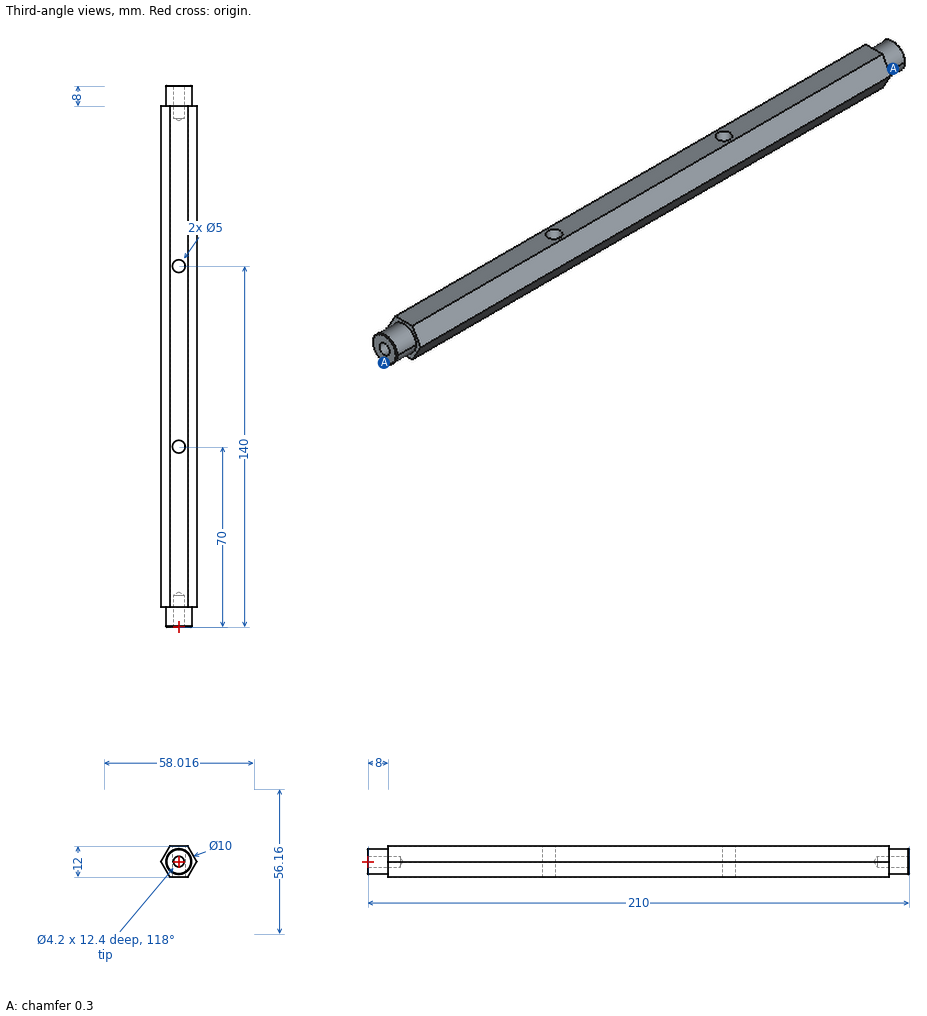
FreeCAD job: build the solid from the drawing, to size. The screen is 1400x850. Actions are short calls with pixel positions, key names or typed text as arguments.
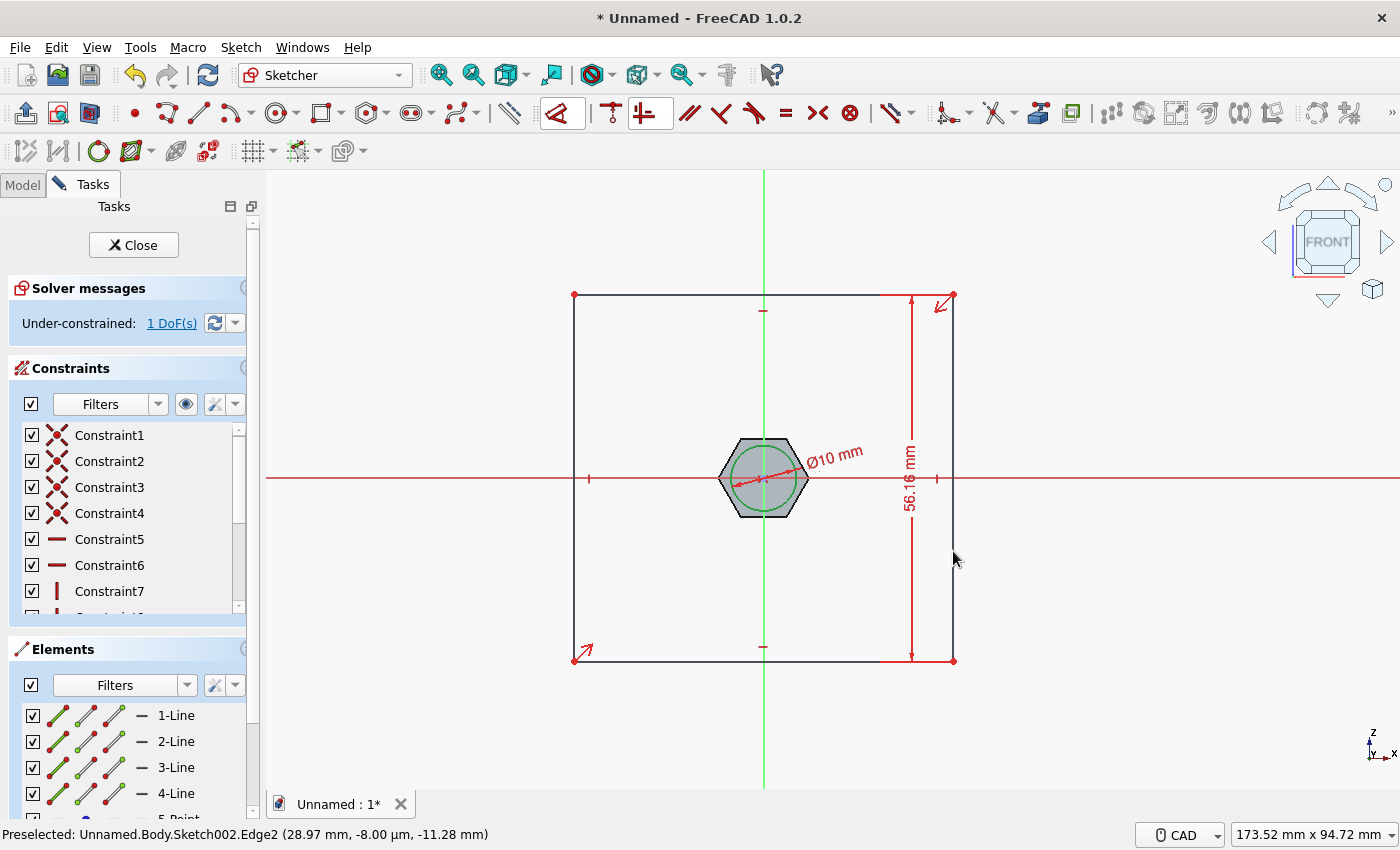
click(688, 662)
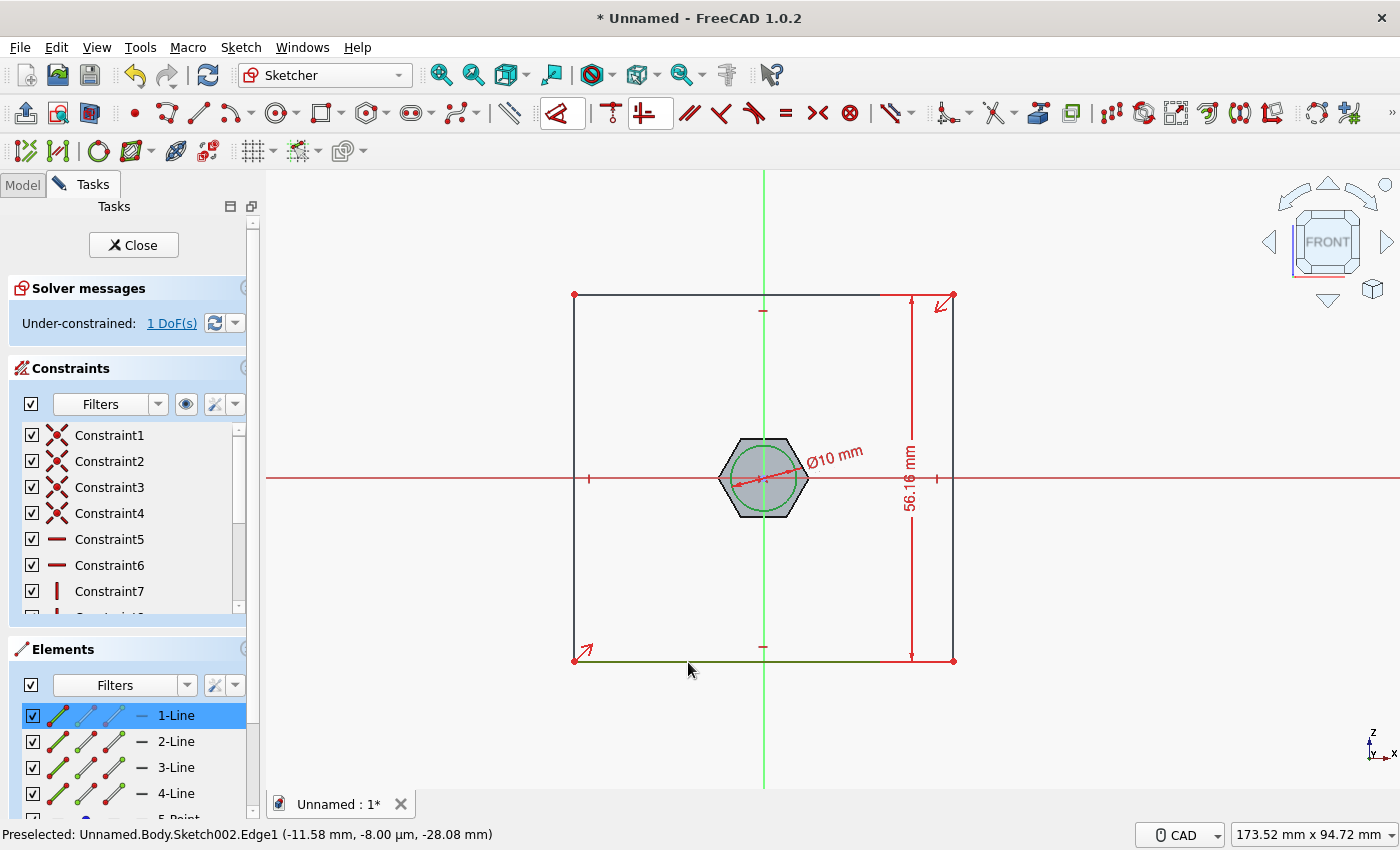
key(l)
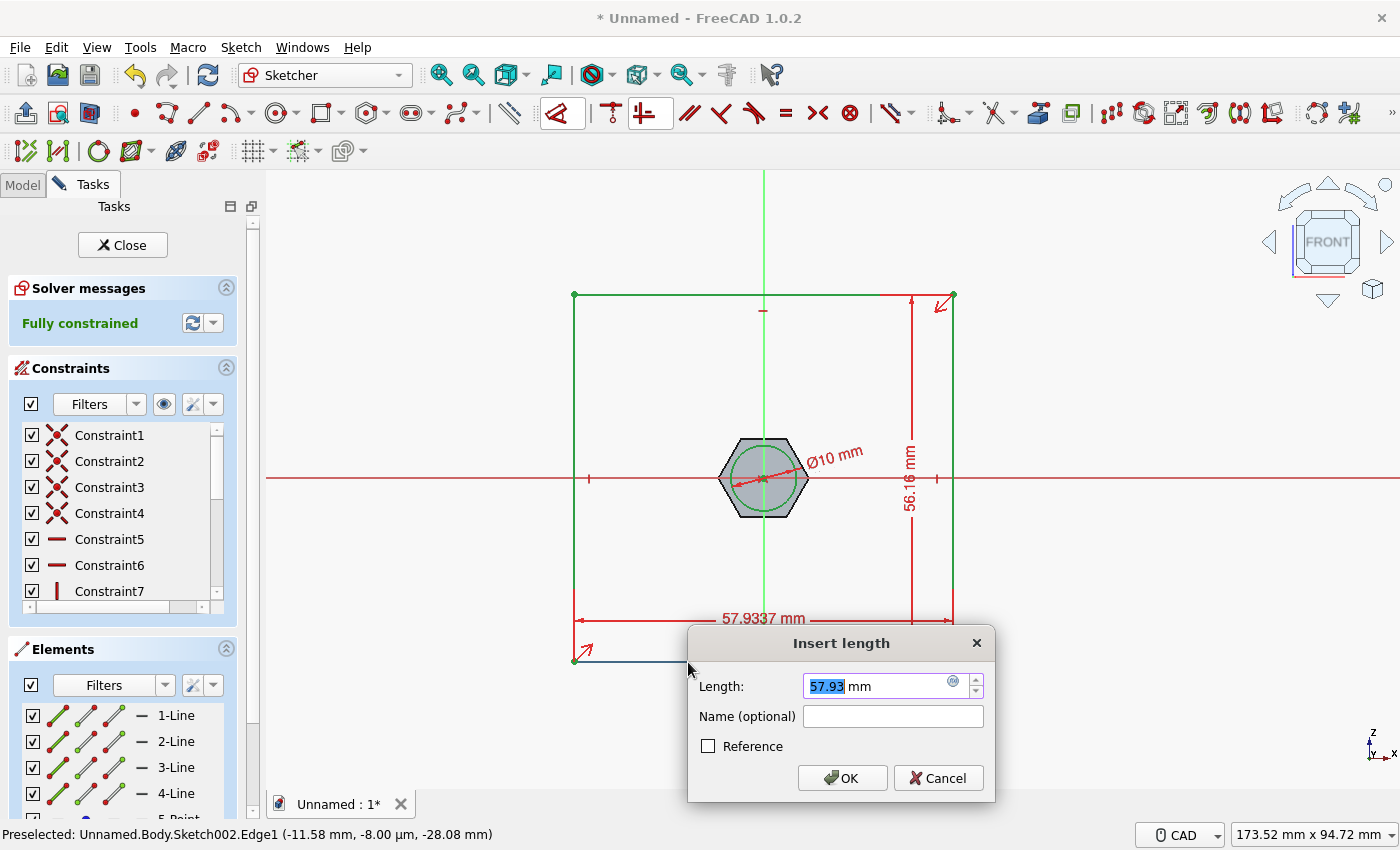
text(58.016)
key(Return)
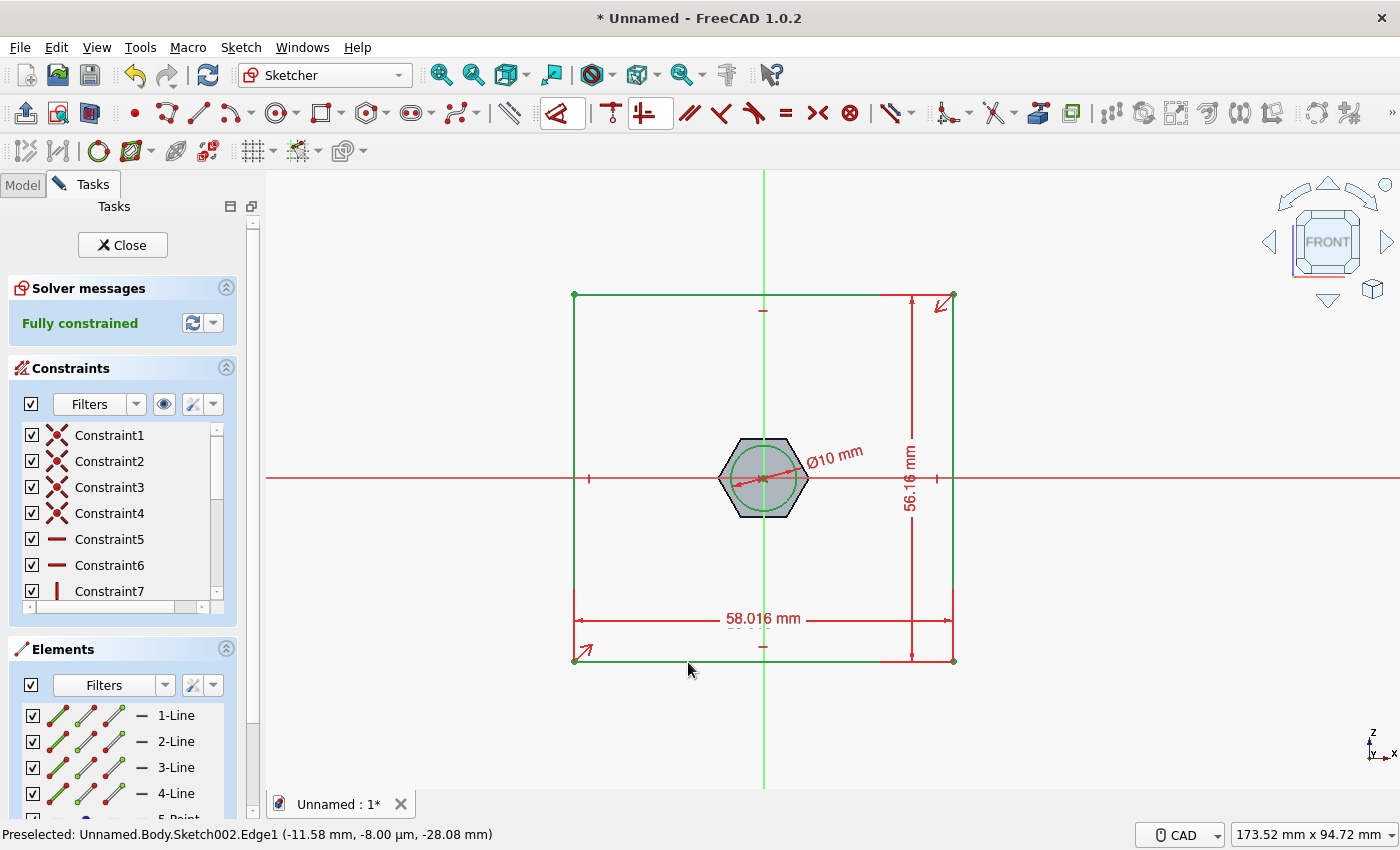
click(123, 245)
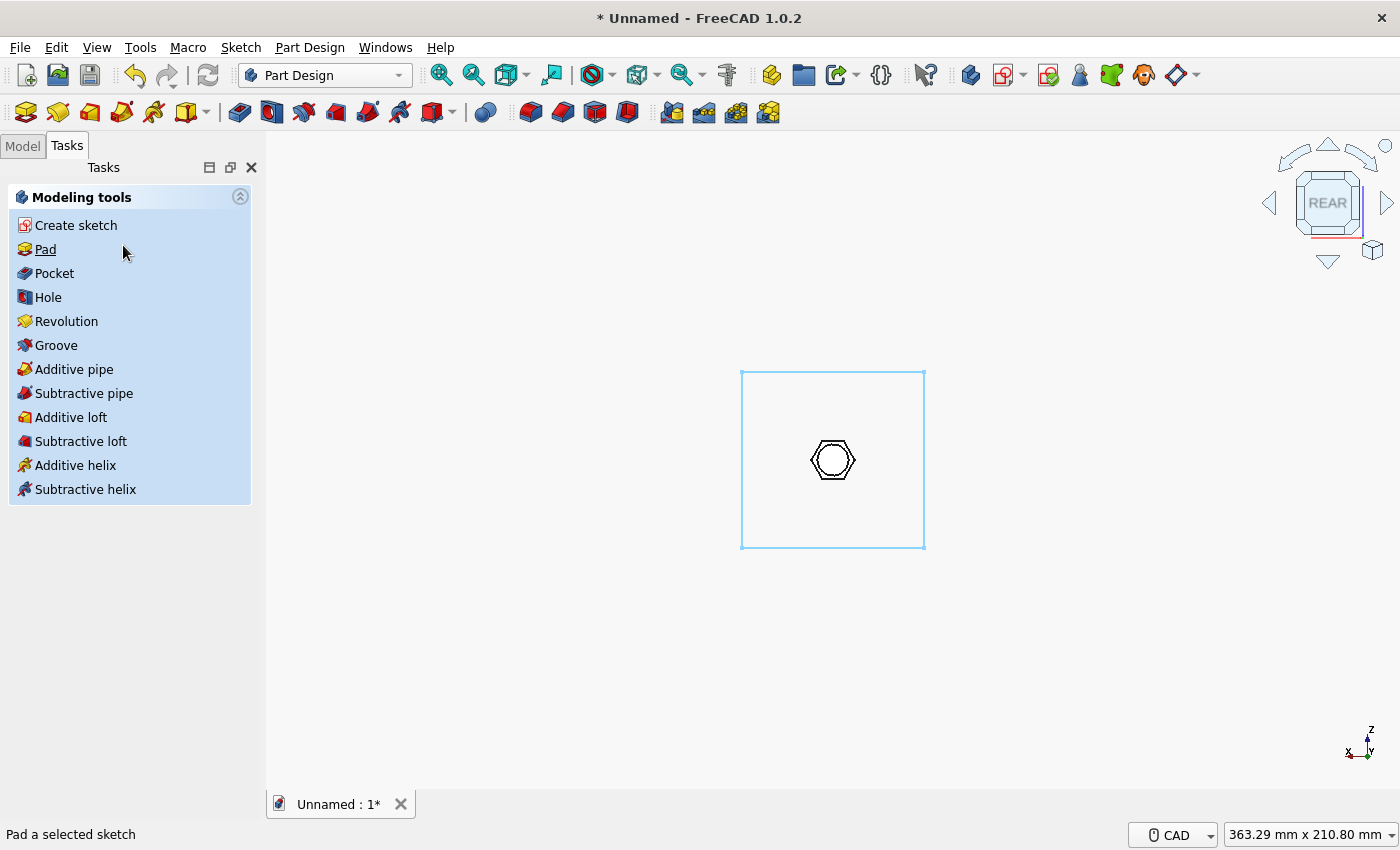
click(240, 112)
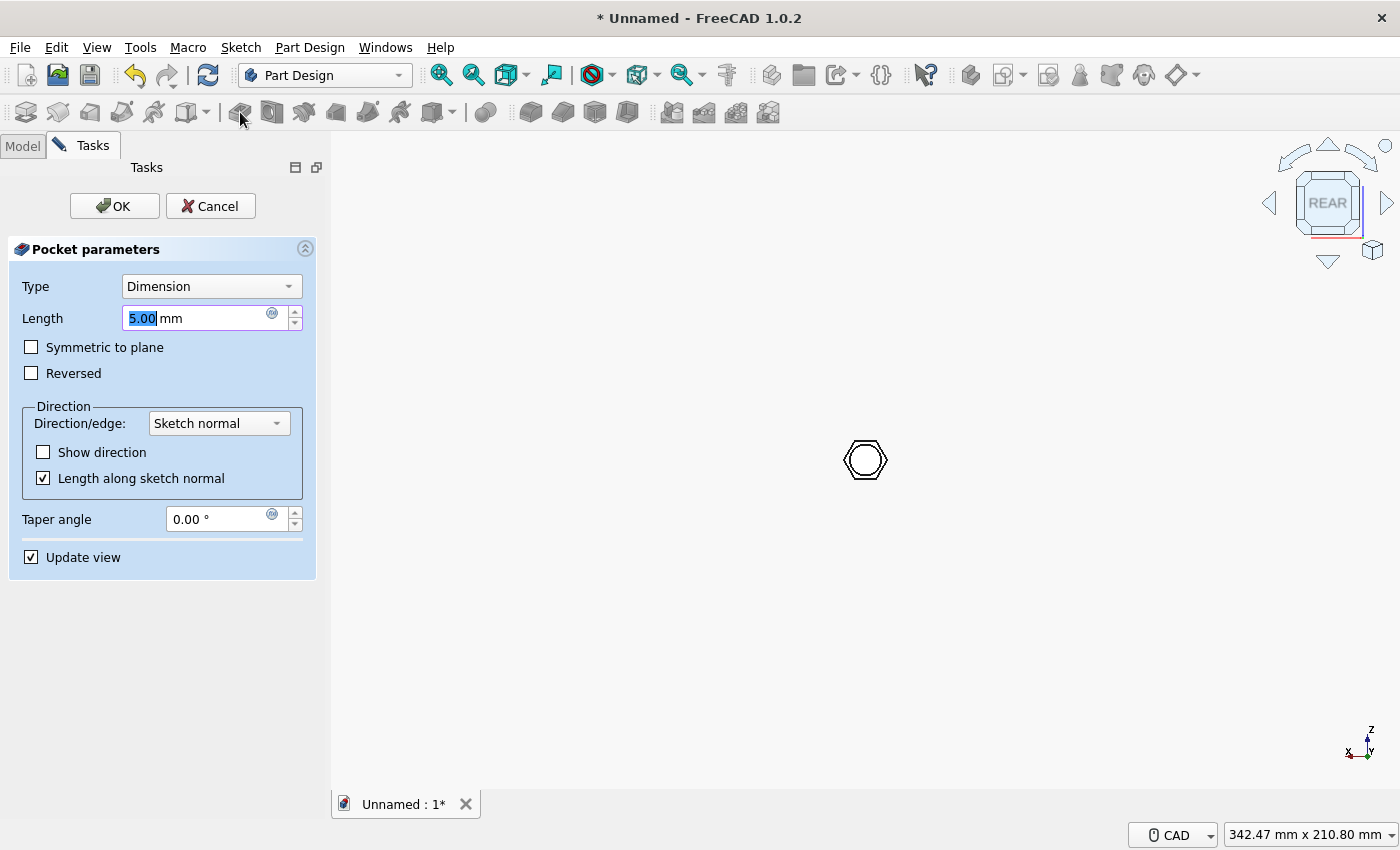
text(8)
key(Tab)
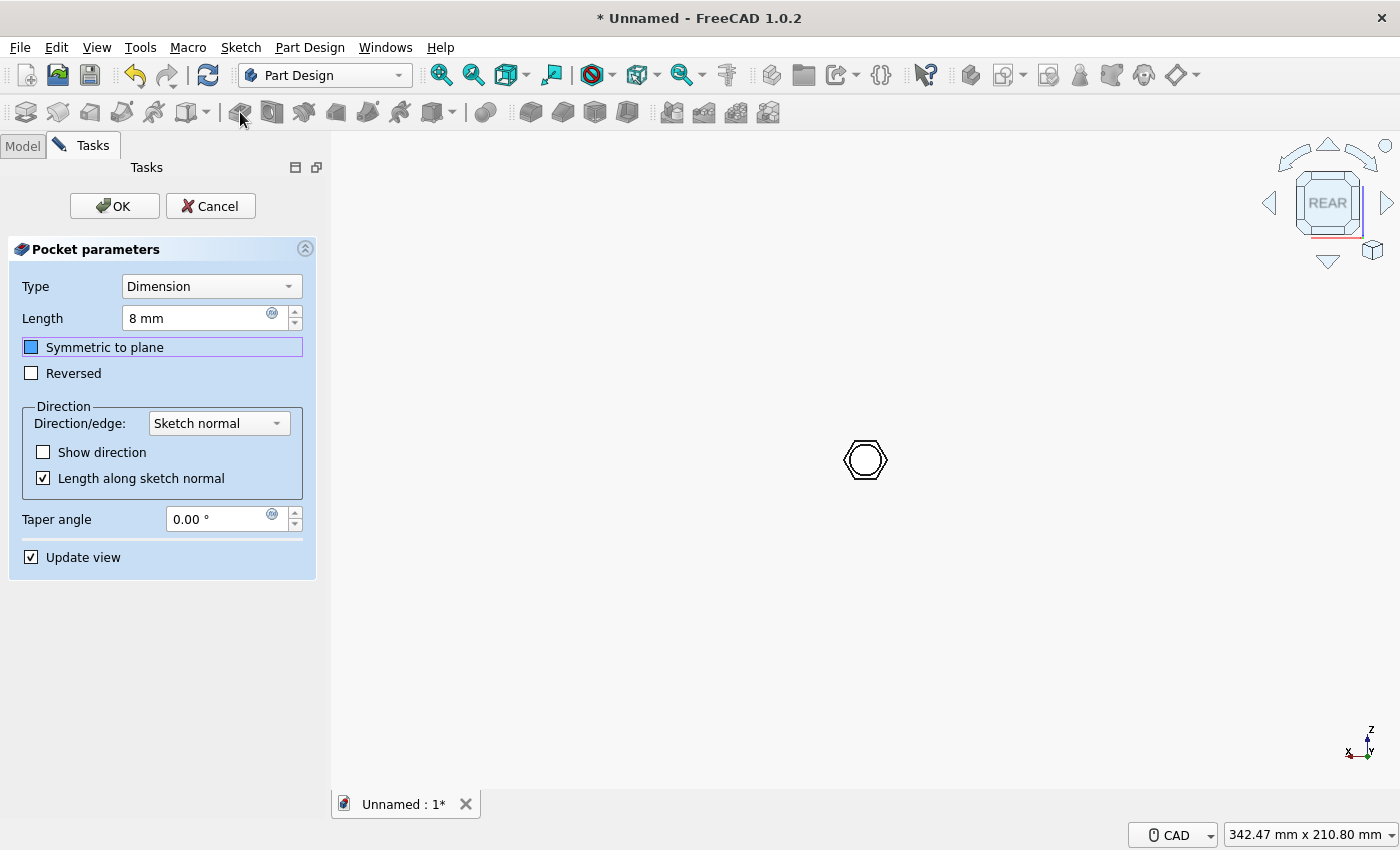
click(115, 206)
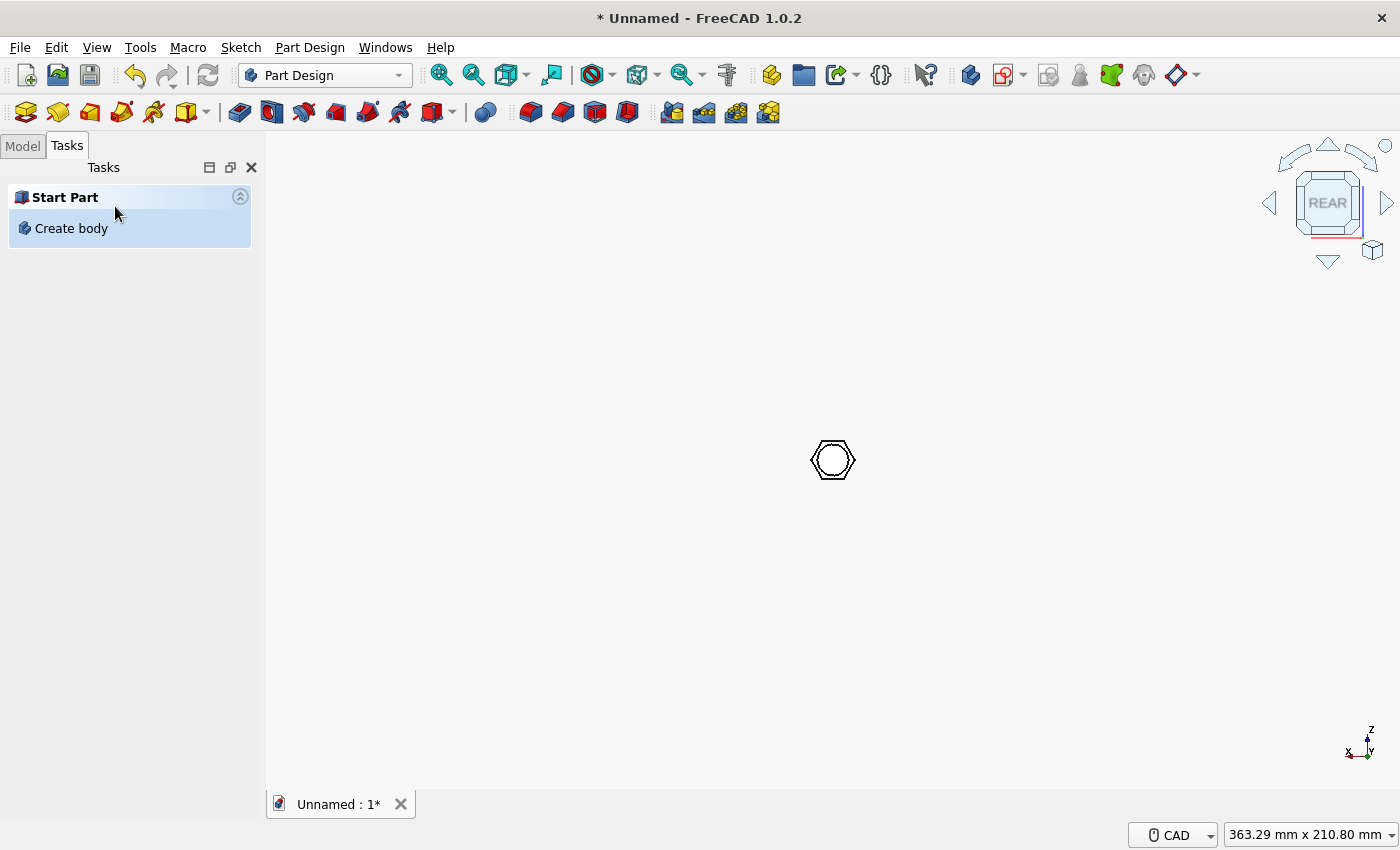
key(v)
key(f)